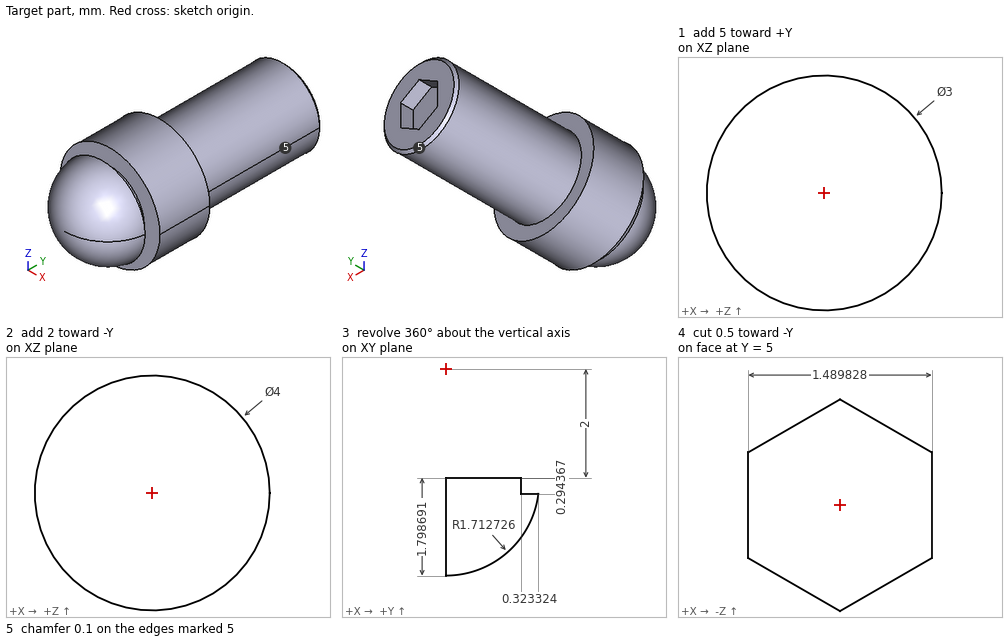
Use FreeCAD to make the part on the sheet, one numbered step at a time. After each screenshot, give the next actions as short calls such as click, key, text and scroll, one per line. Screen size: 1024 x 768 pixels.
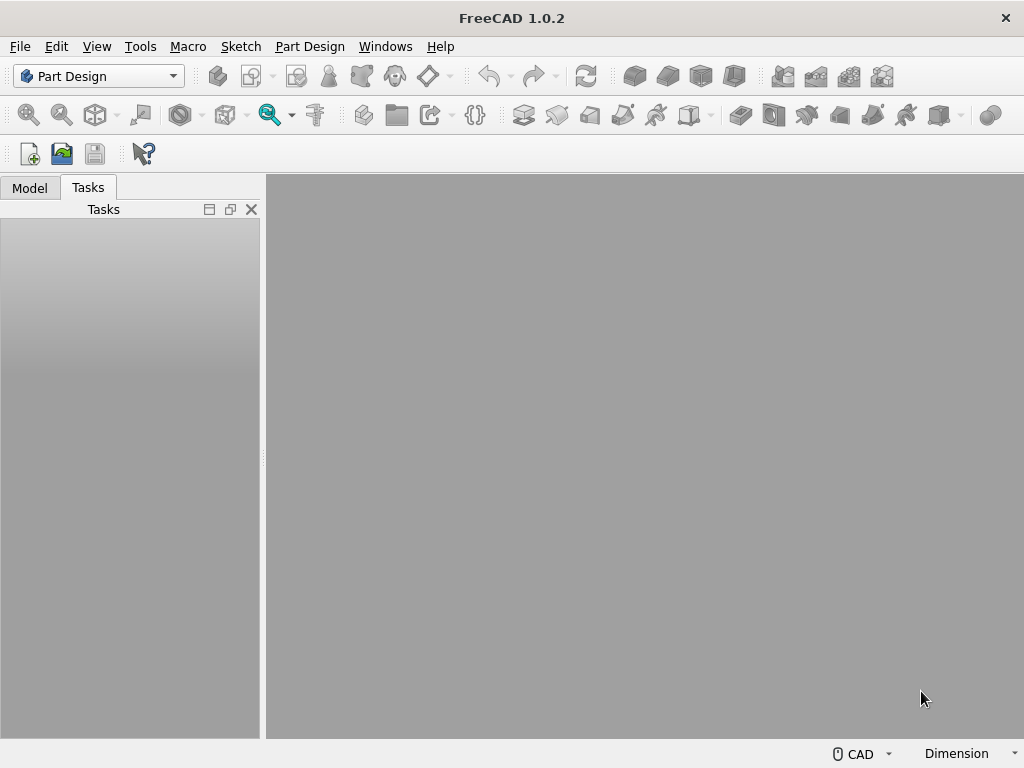
click(29, 154)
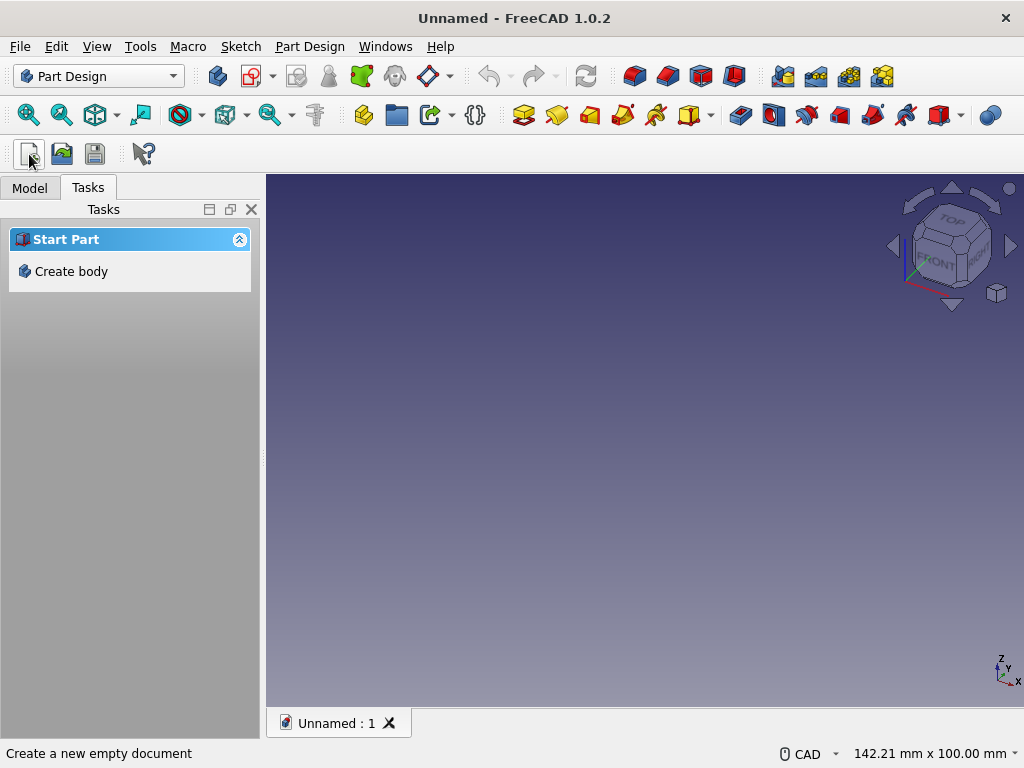
click(250, 76)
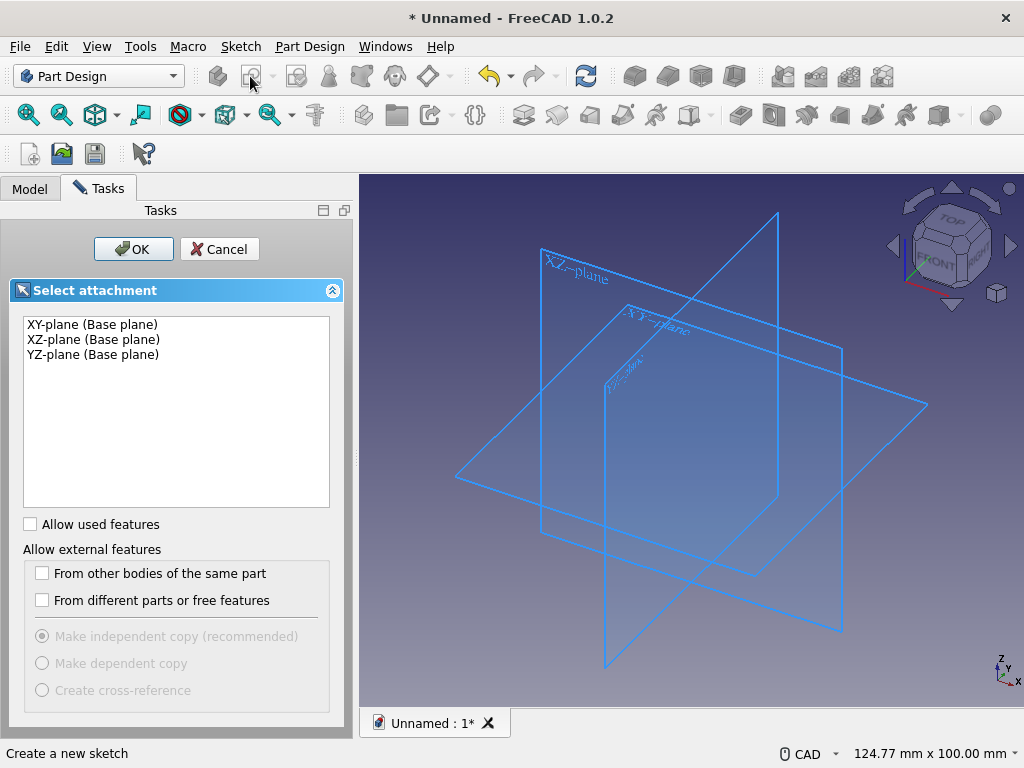
click(84, 340)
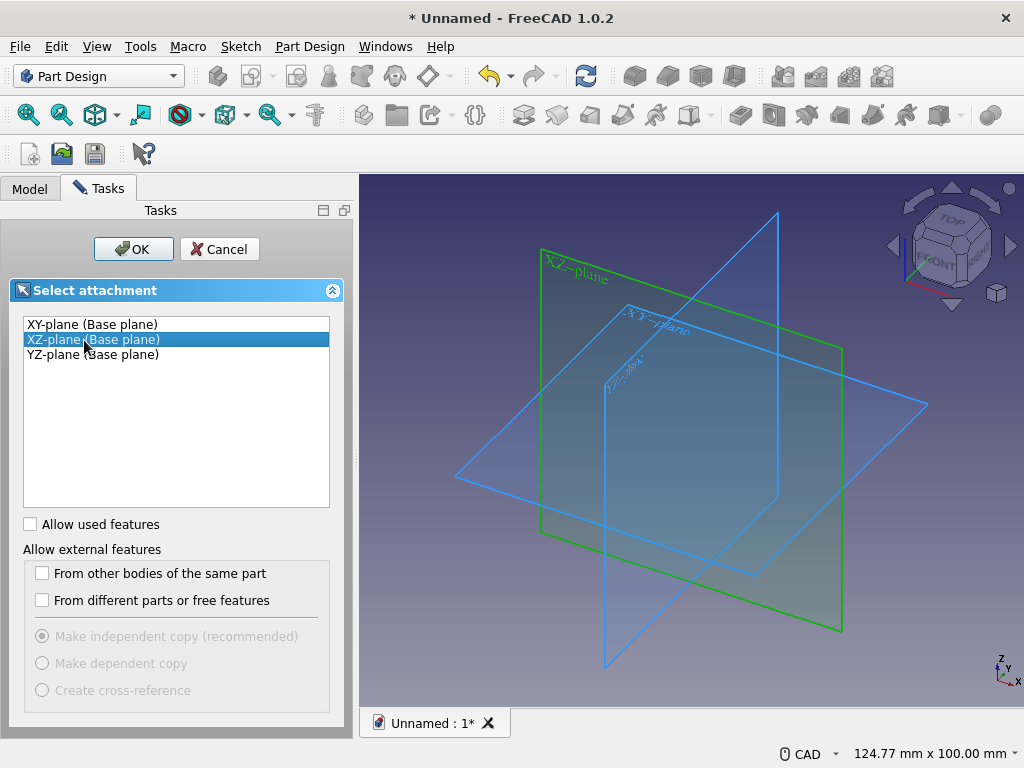
click(134, 249)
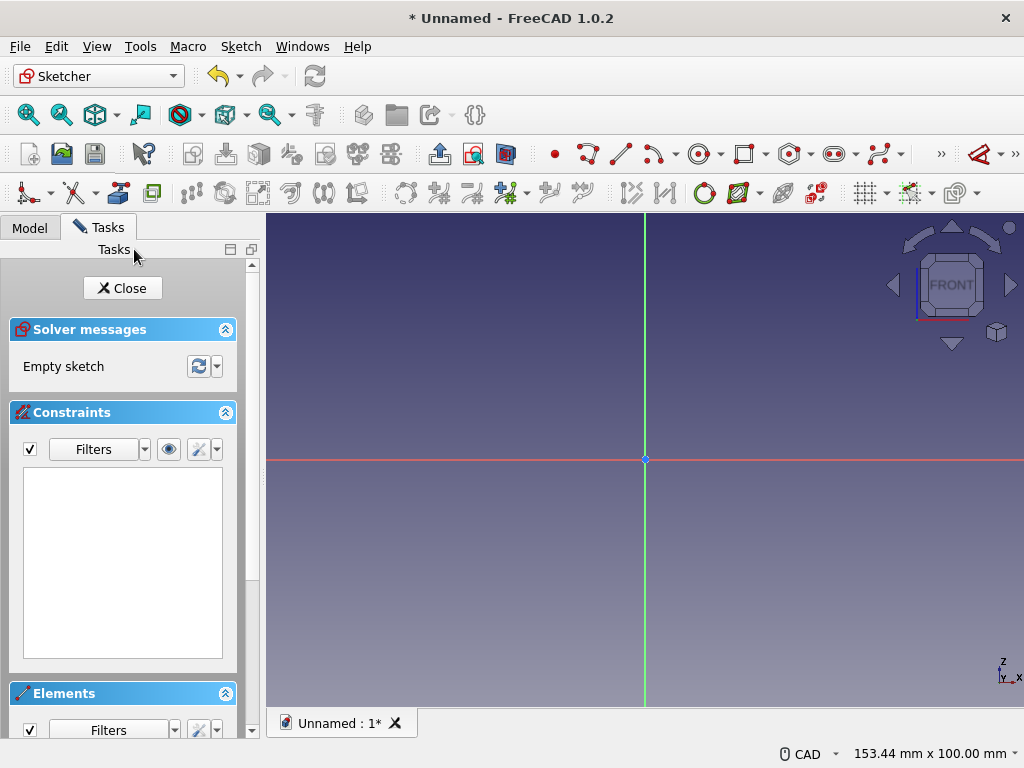
scroll(649, 460, up, 15)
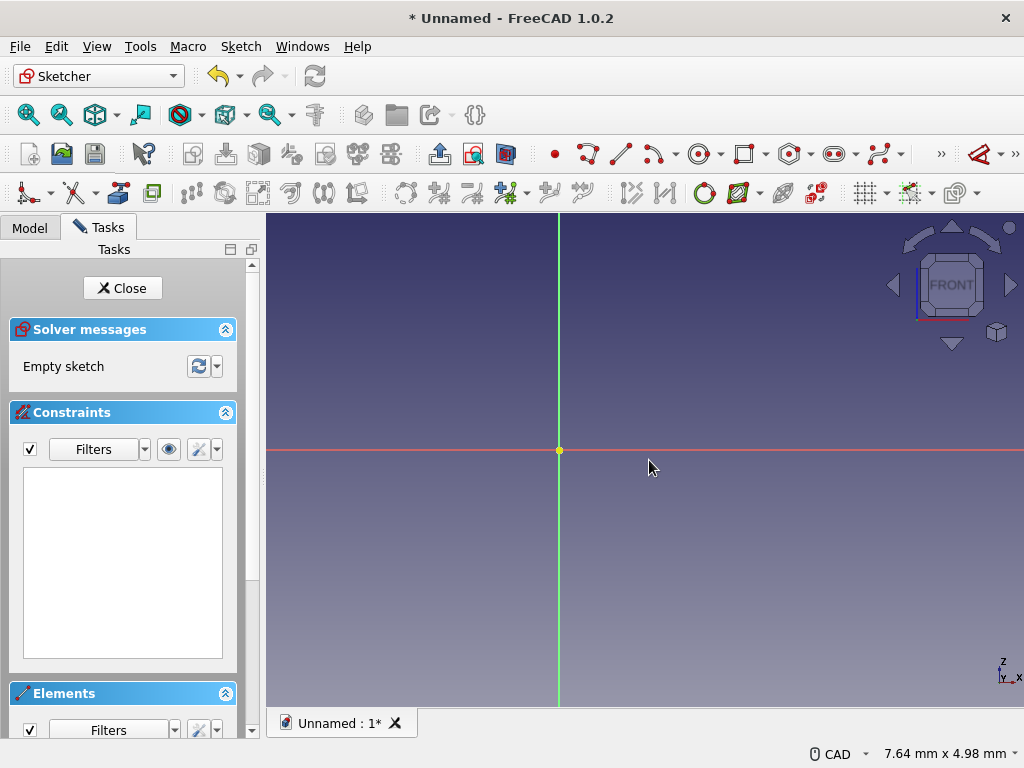
click(698, 154)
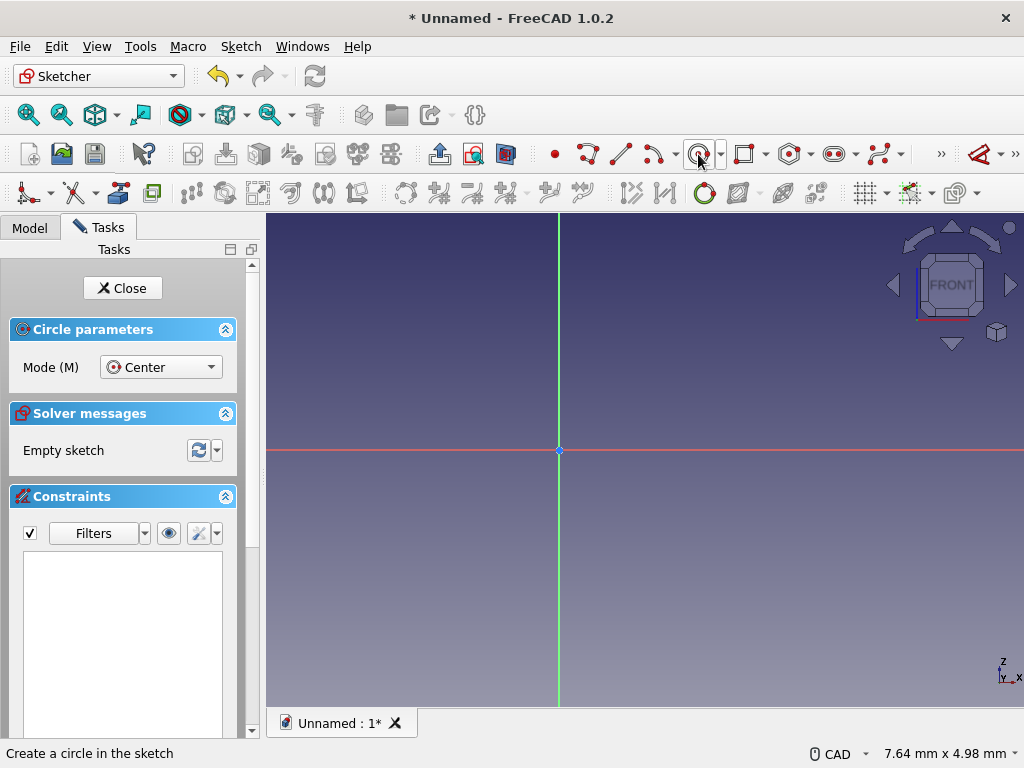
click(559, 450)
click(664, 345)
key(Escape)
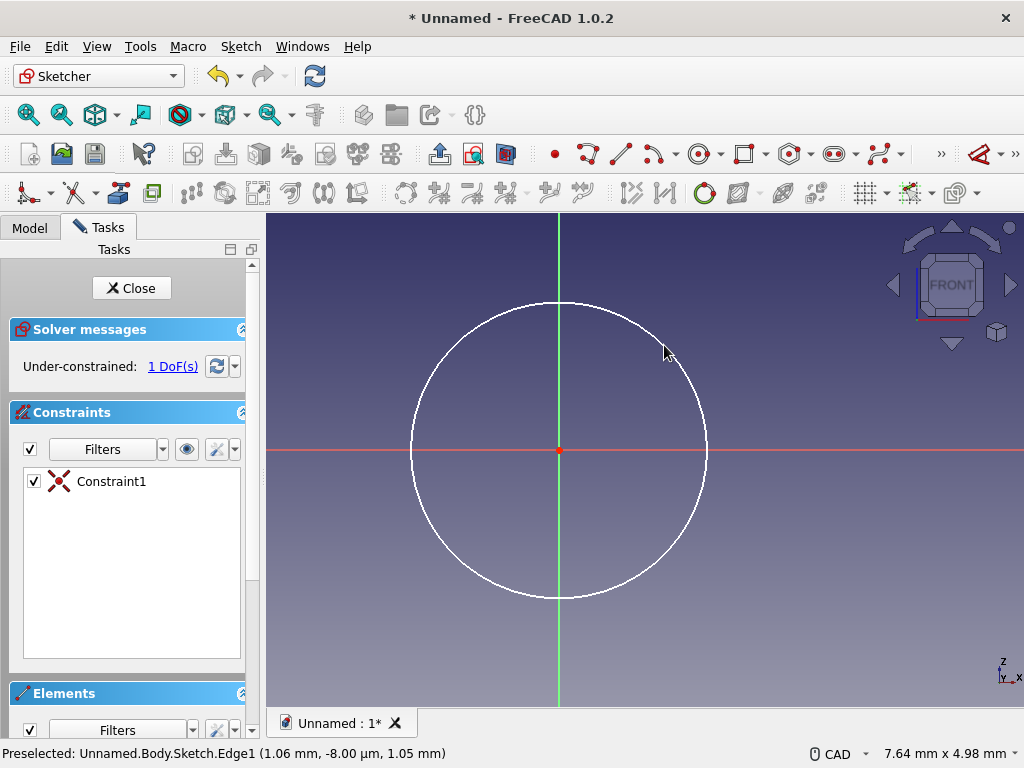
click(663, 345)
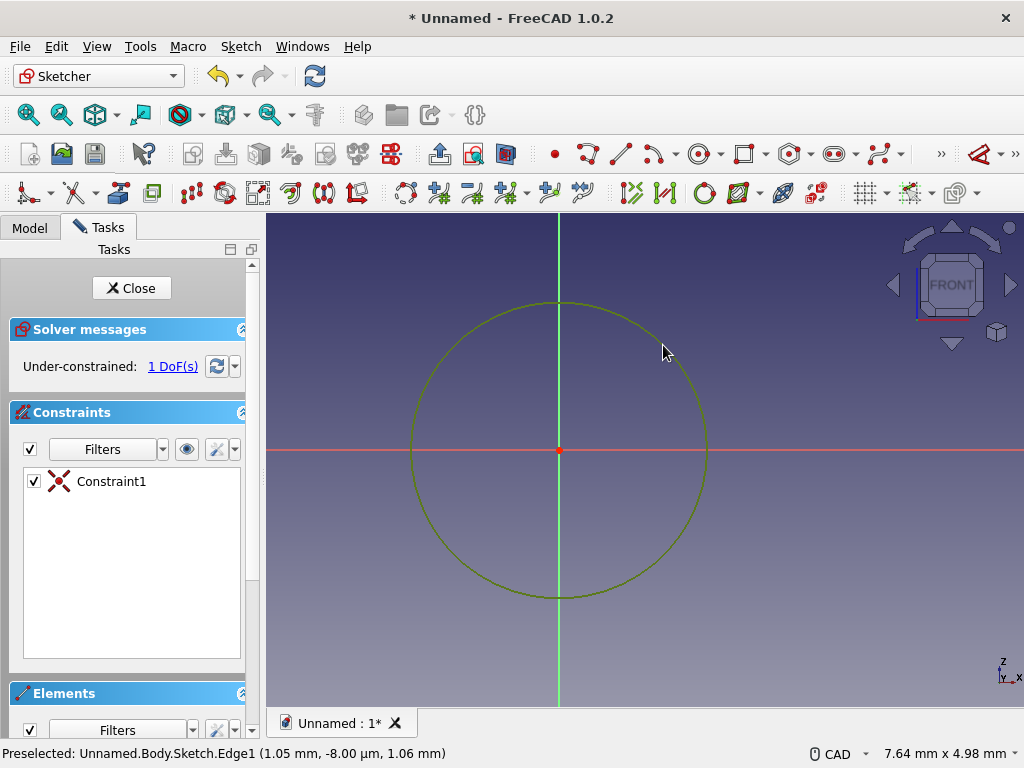
key(k)
key(o)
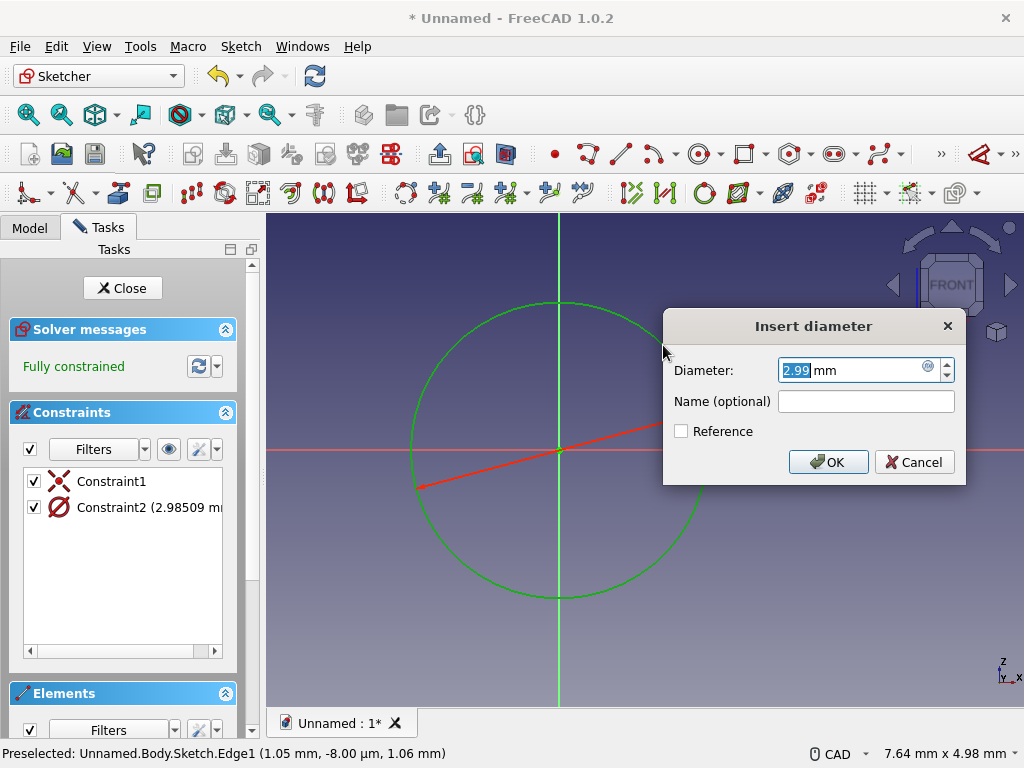
text(3)
key(Return)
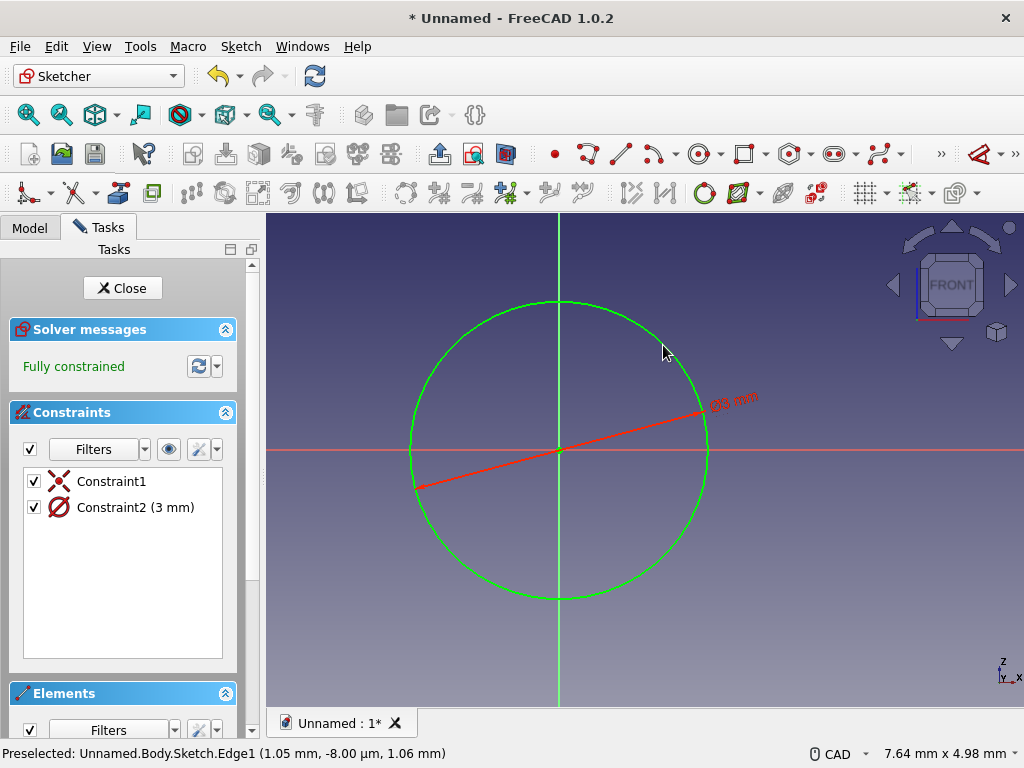
click(123, 288)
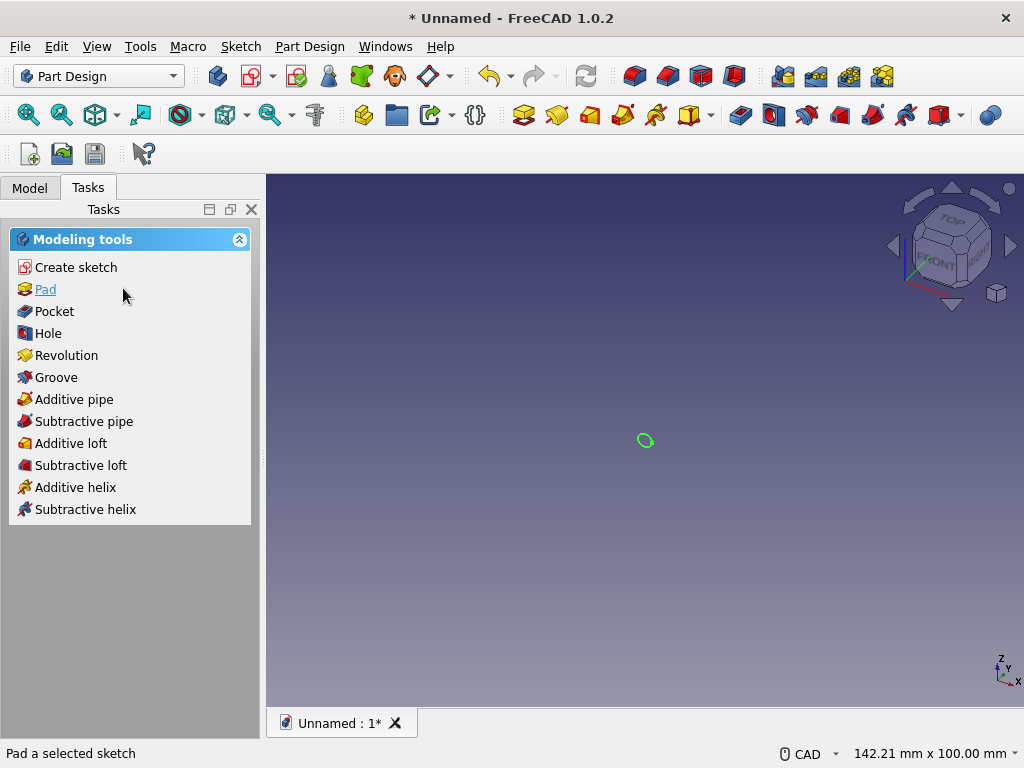
click(524, 116)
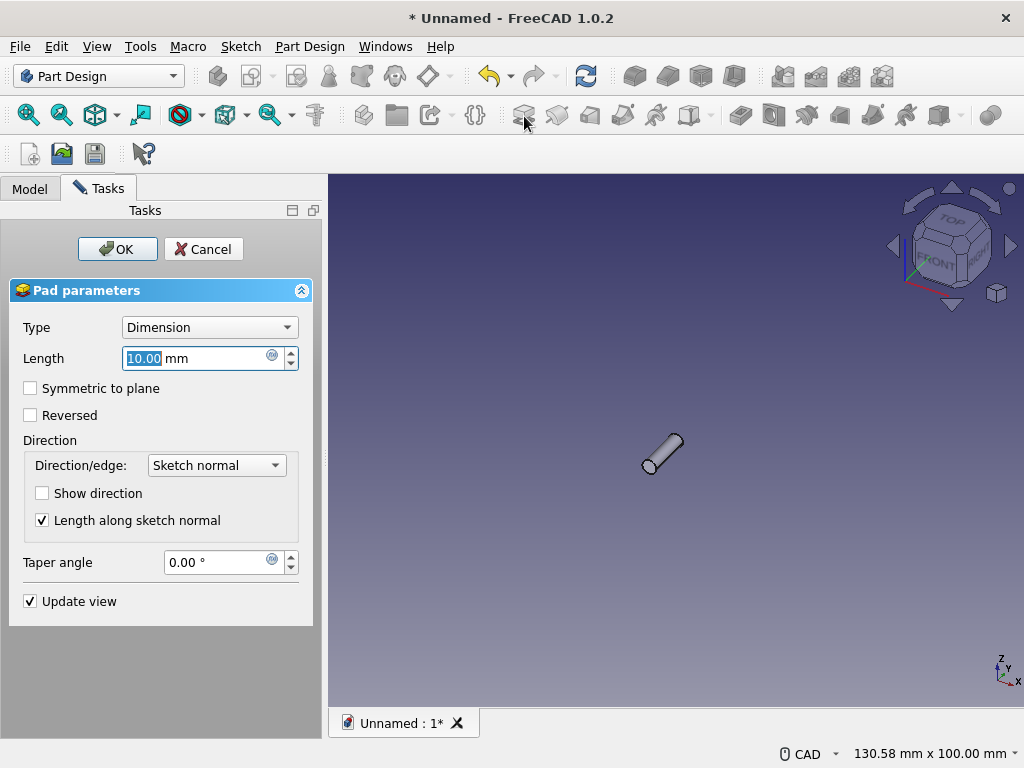
text(5)
key(Tab)